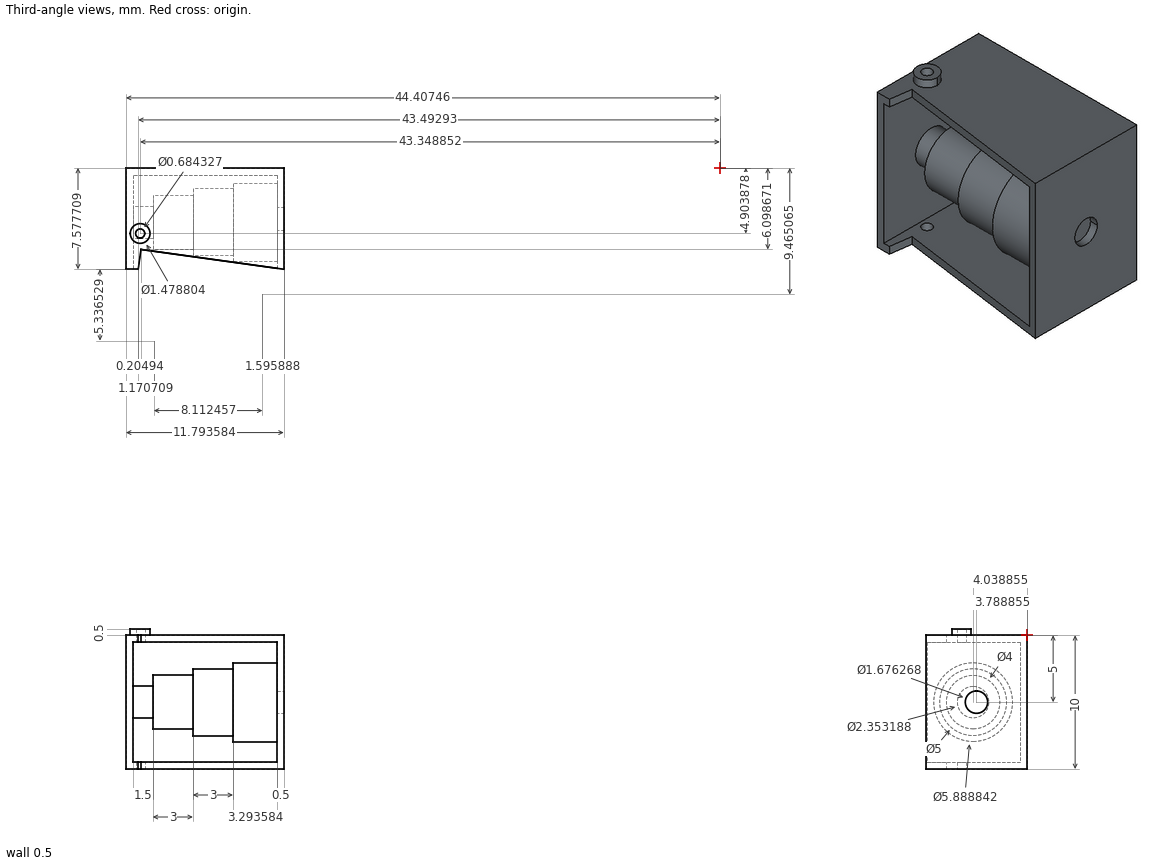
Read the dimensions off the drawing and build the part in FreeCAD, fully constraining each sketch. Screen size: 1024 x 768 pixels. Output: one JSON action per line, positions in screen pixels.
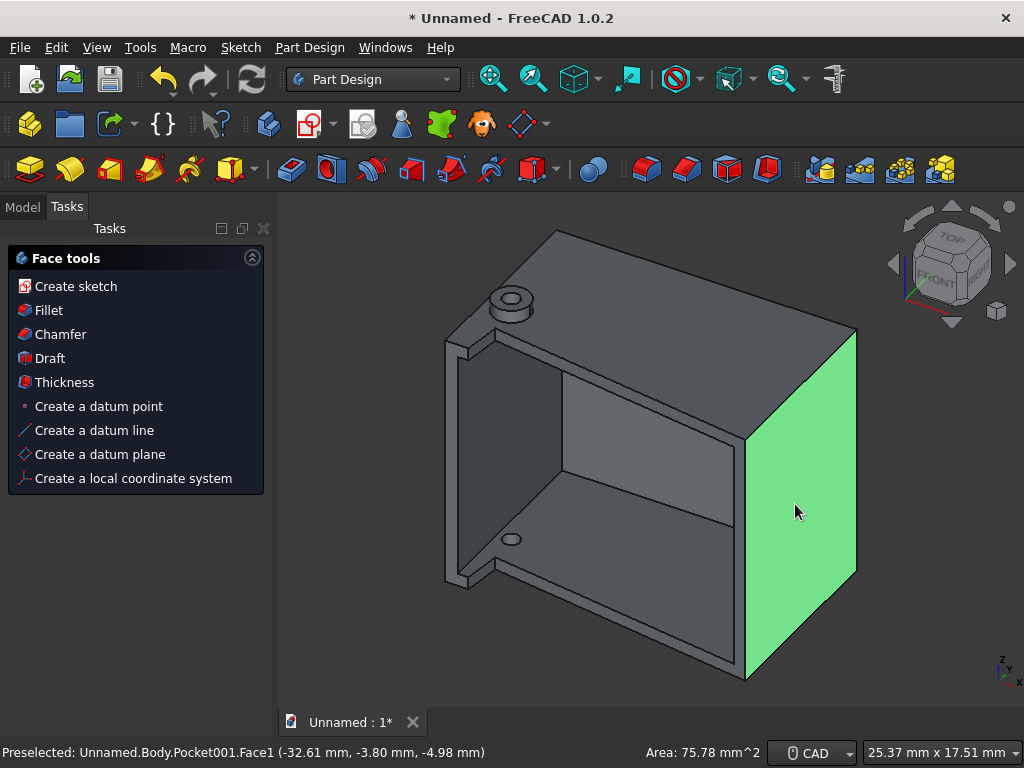
{"action": "left_click", "coordinate": [310, 124]}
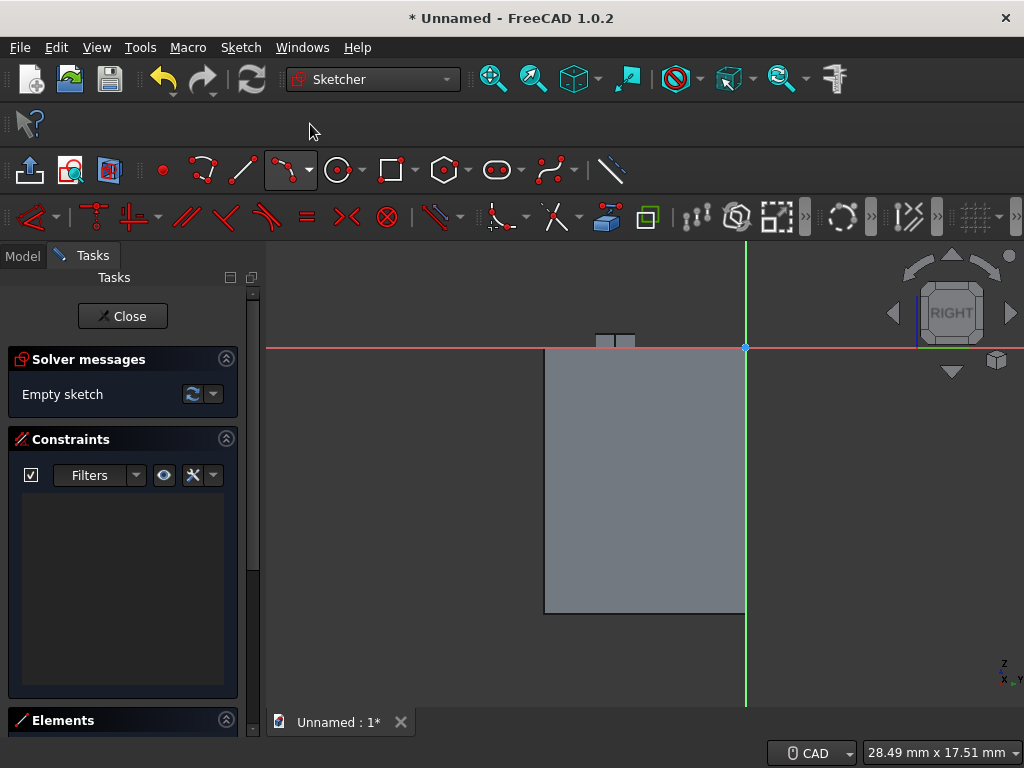
{"action": "scroll", "coordinate": [659, 482], "scroll_direction": "up", "scroll_amount": 9}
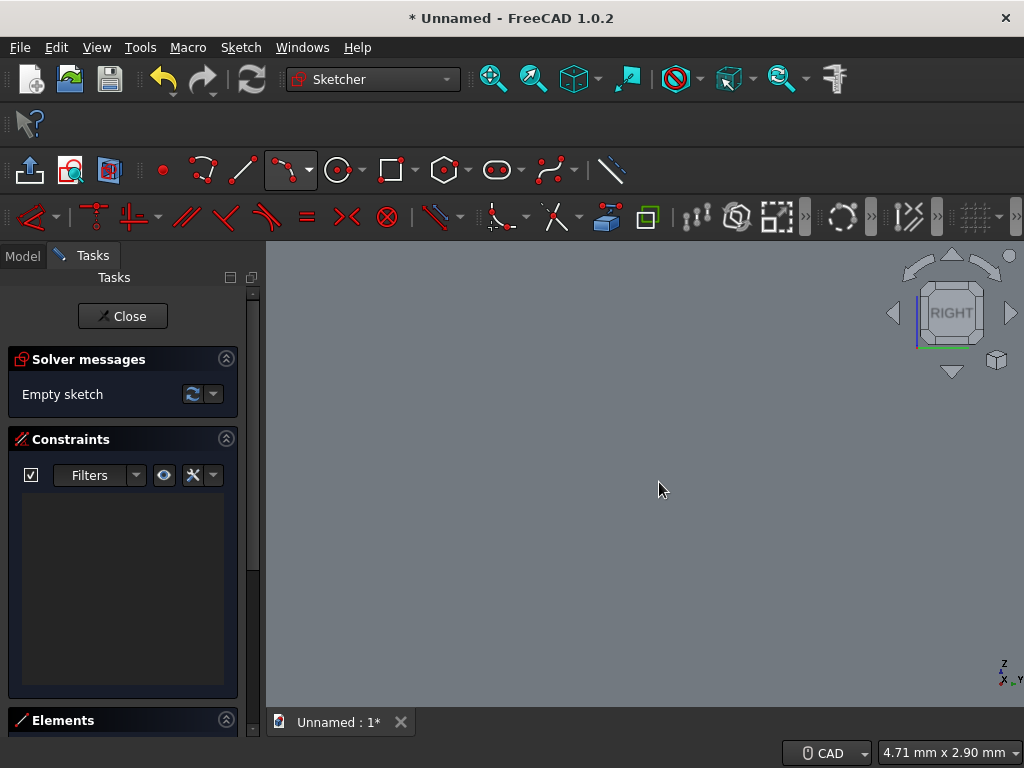
{"action": "left_click", "coordinate": [338, 170]}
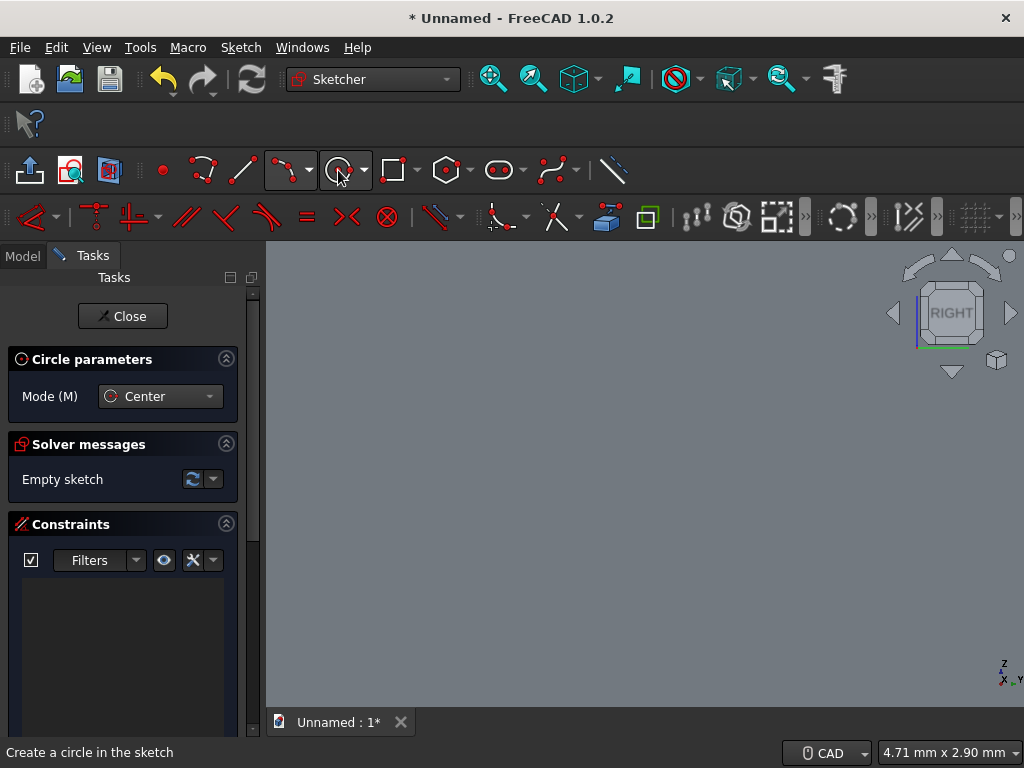
{"action": "left_click", "coordinate": [572, 471]}
{"action": "left_click", "coordinate": [667, 376]}
{"action": "key", "text": "Escape"}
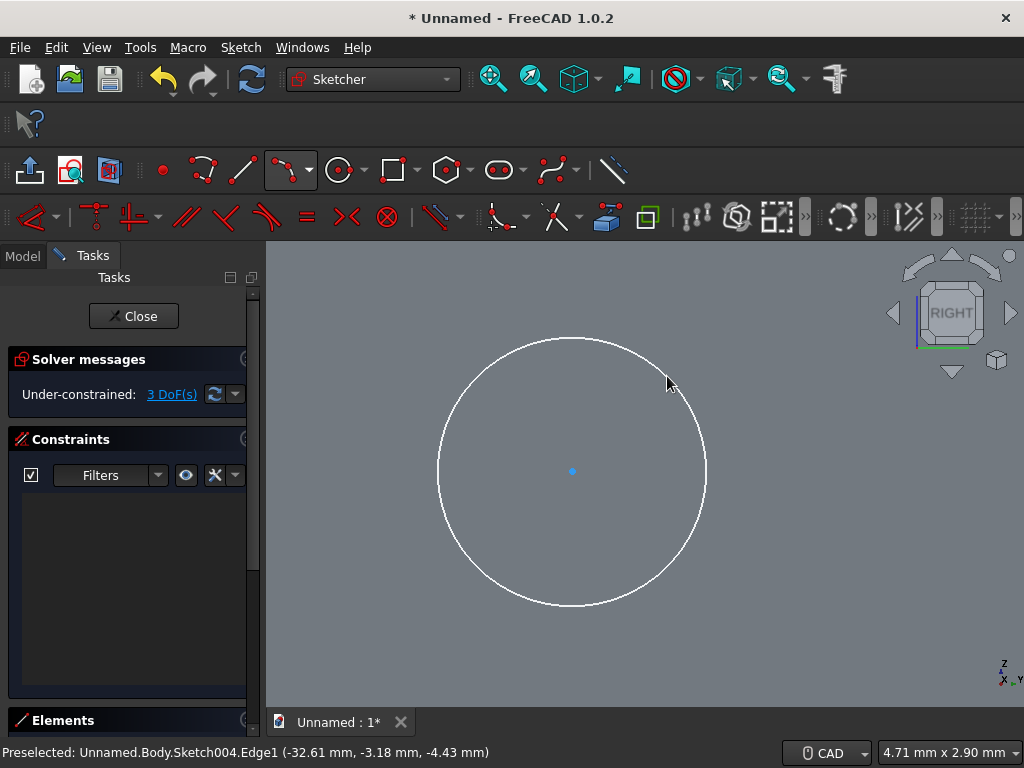
{"action": "left_click", "coordinate": [32, 218]}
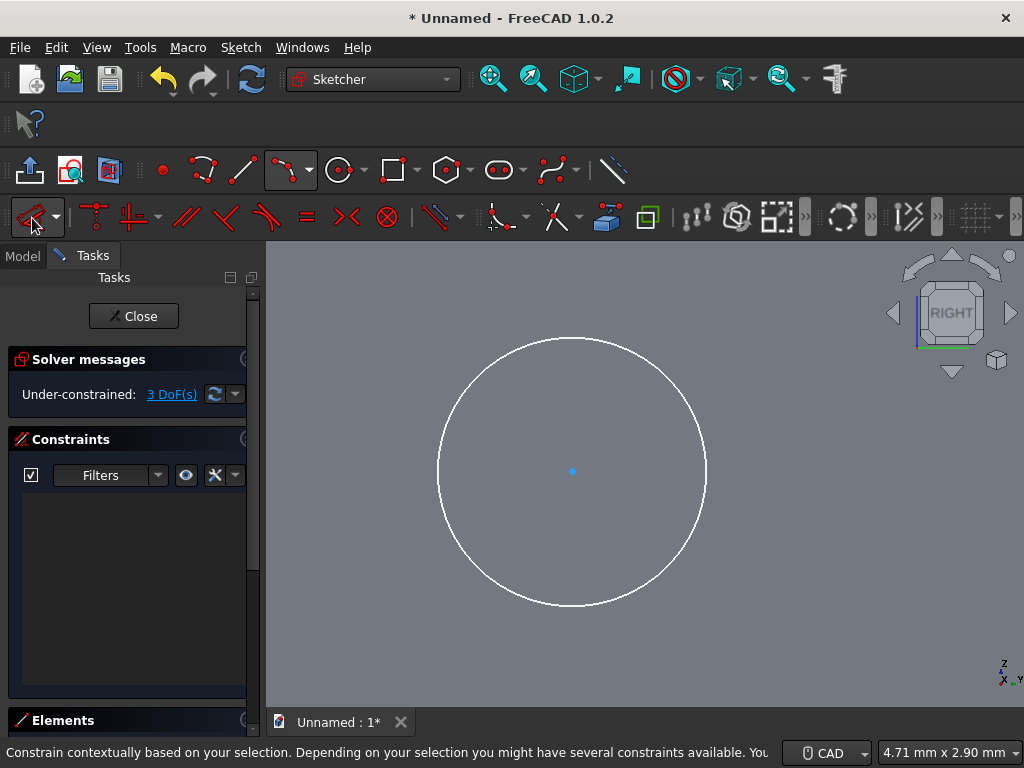
{"action": "left_click", "coordinate": [667, 377]}
{"action": "left_click", "coordinate": [690, 354]}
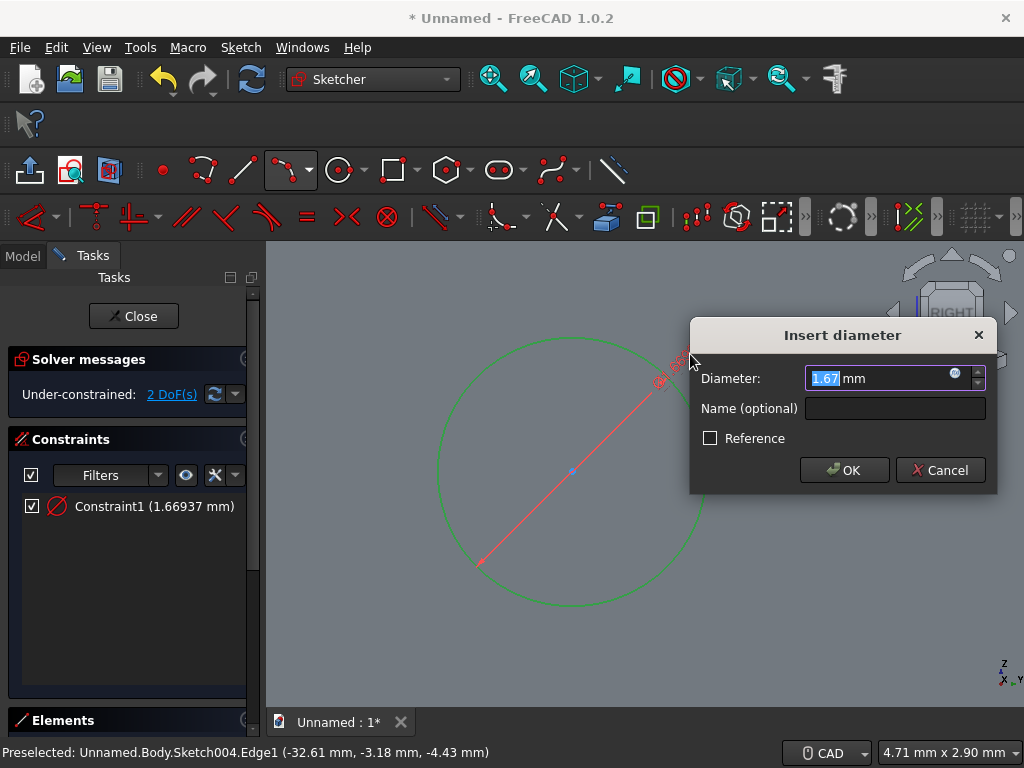
{"action": "type", "text": "1.676268"}
{"action": "key", "text": "Return"}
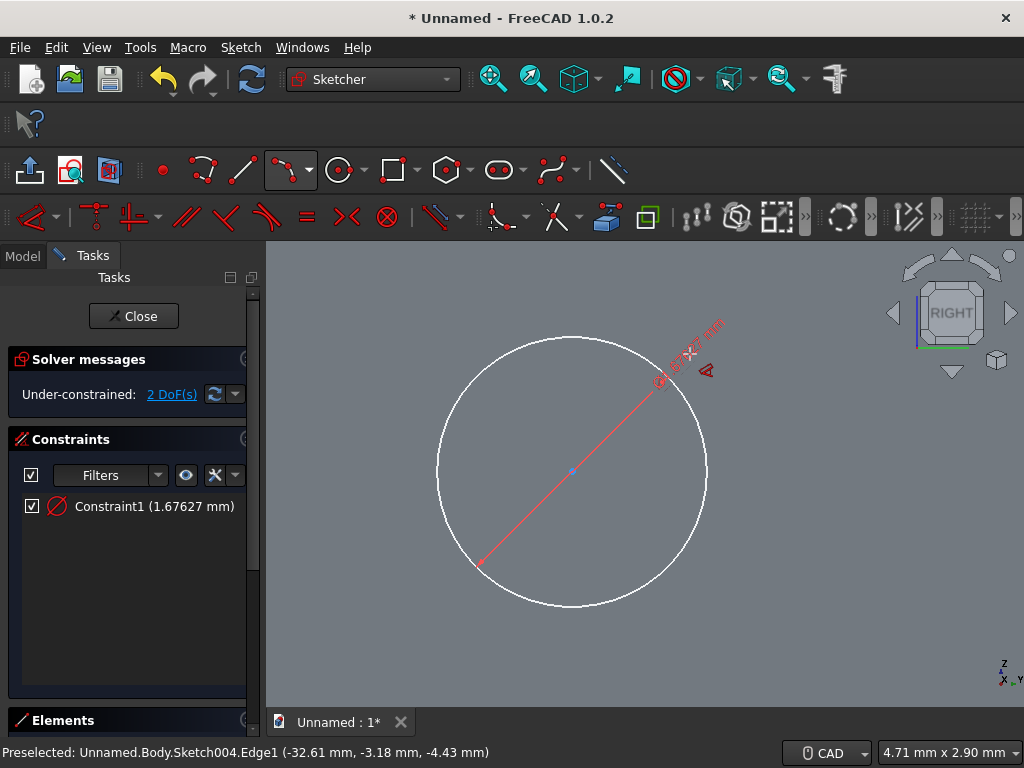
{"action": "left_click", "coordinate": [572, 472]}
{"action": "left_click", "coordinate": [538, 371]}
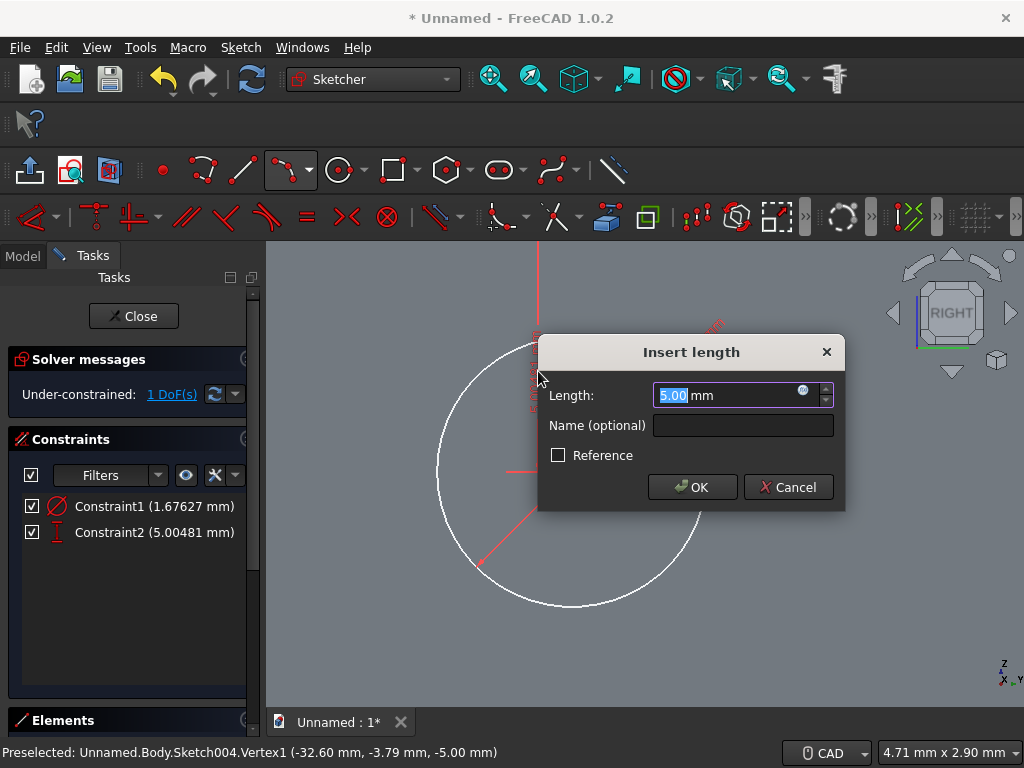
{"action": "type", "text": "5"}
{"action": "key", "text": "Return"}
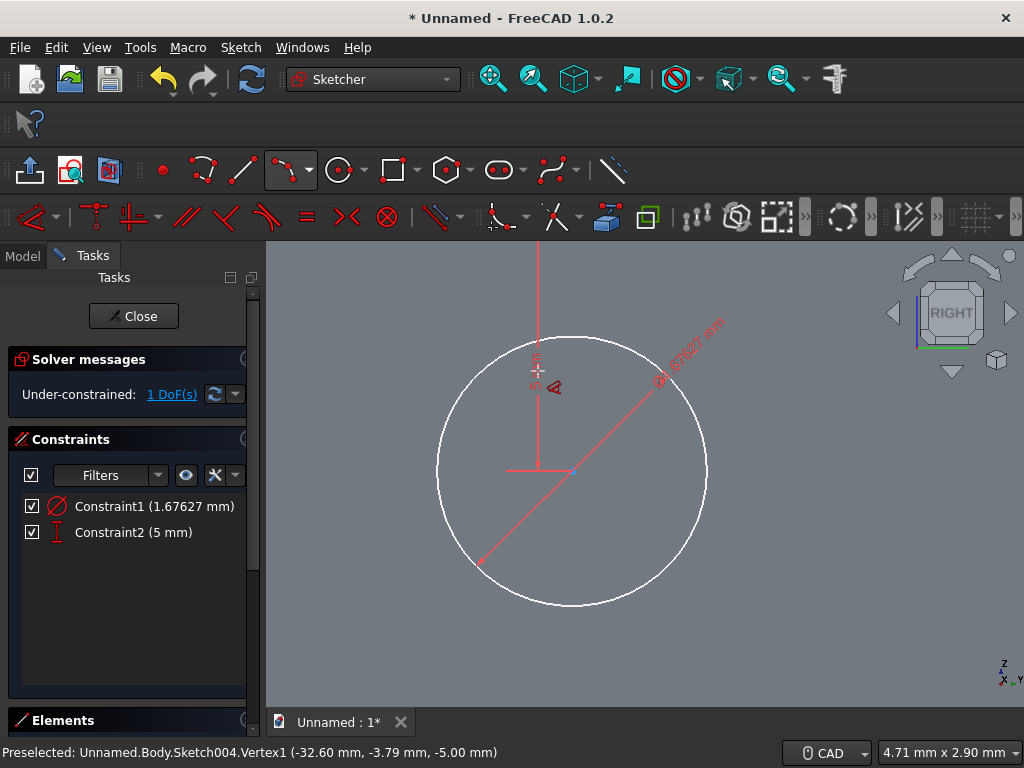
{"action": "left_click", "coordinate": [572, 471]}
{"action": "left_click", "coordinate": [649, 505]}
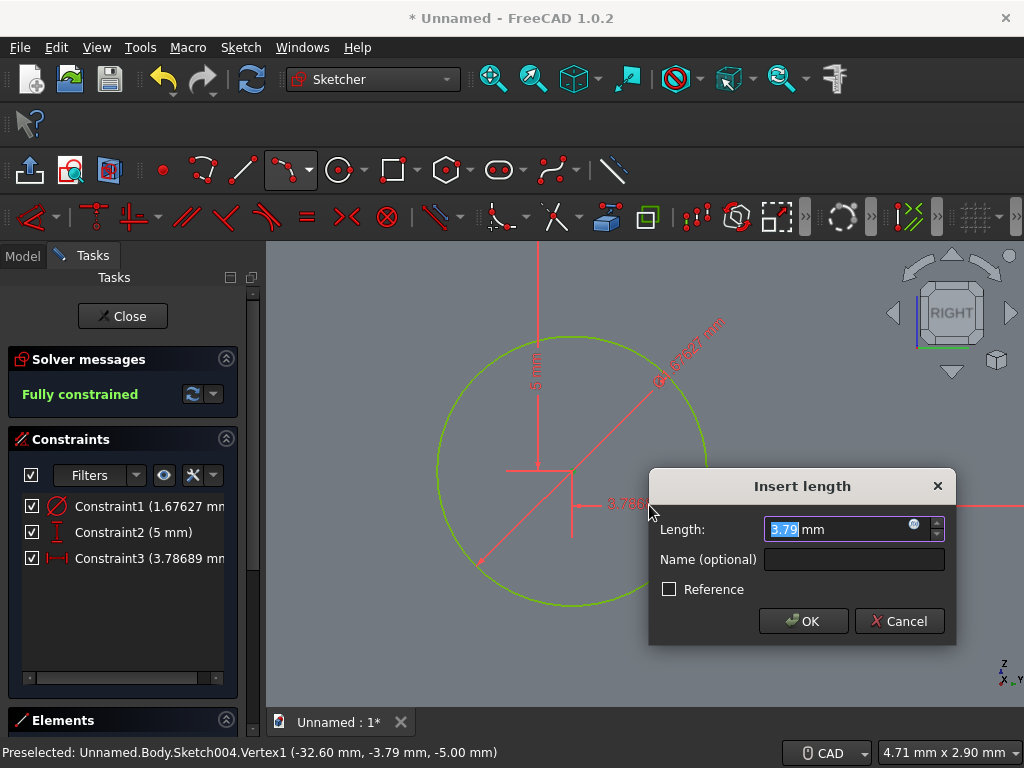
{"action": "type", "text": "3.788855"}
{"action": "key", "text": "Return"}
{"action": "key", "text": "Escape"}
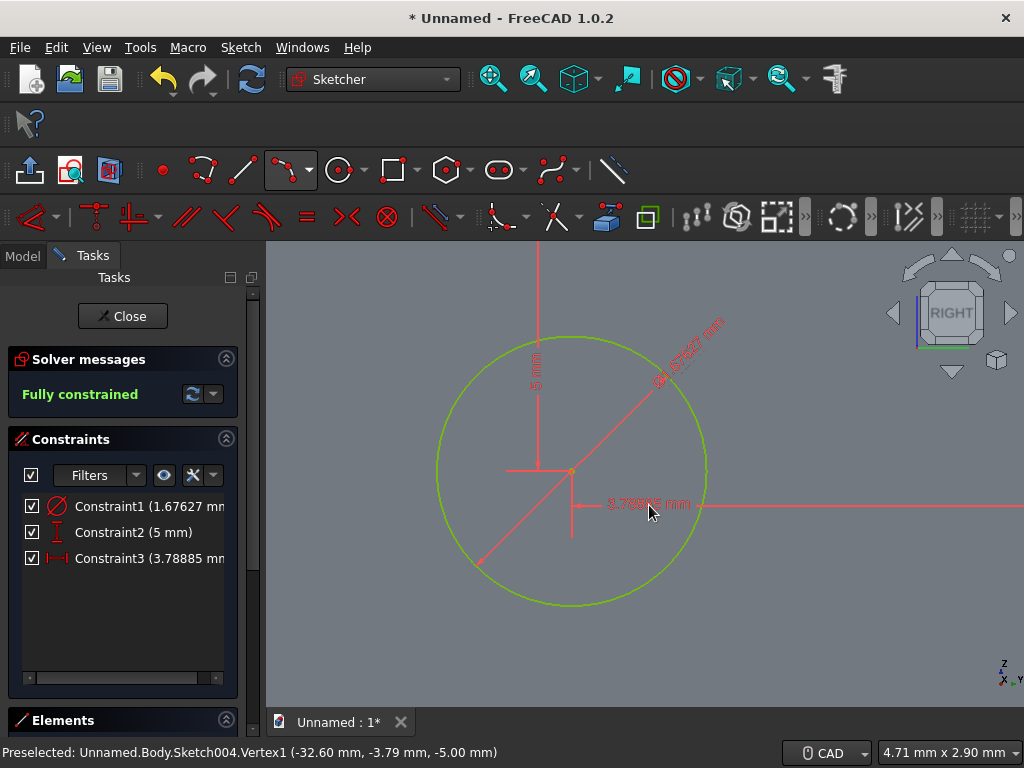
{"action": "left_click", "coordinate": [123, 316]}